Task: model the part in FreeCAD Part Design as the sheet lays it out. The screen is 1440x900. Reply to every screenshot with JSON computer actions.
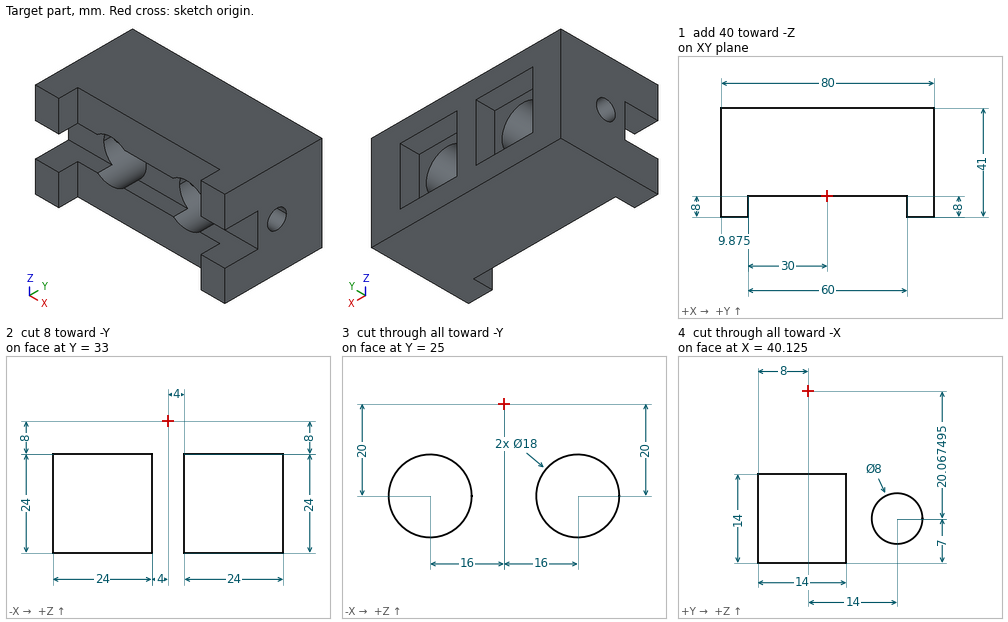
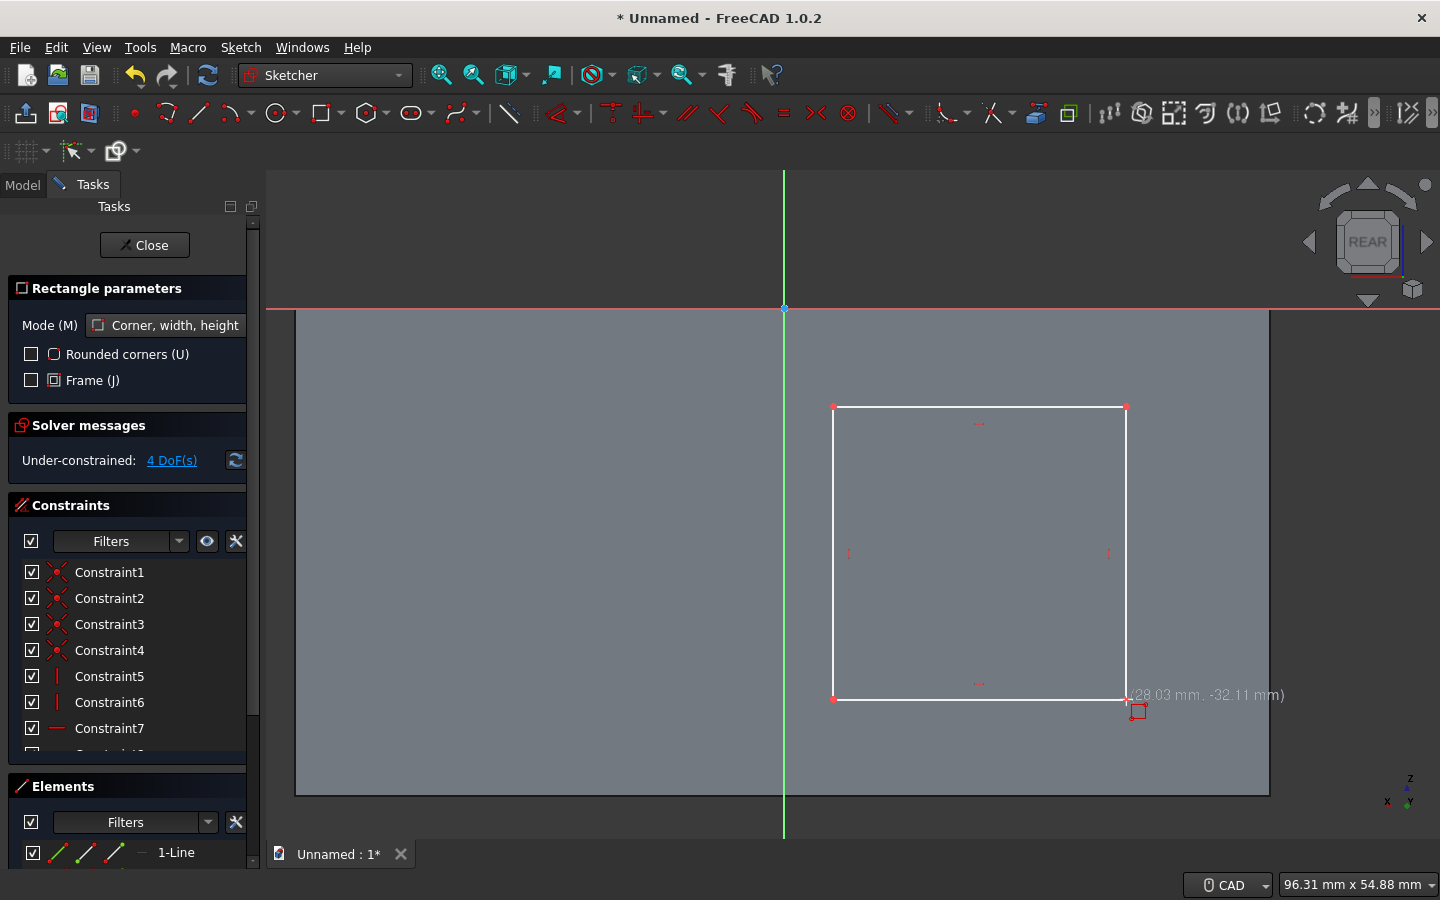
{"action": "left_click", "coordinate": [443, 406]}
{"action": "left_click", "coordinate": [736, 699]}
{"action": "key", "text": "Escape"}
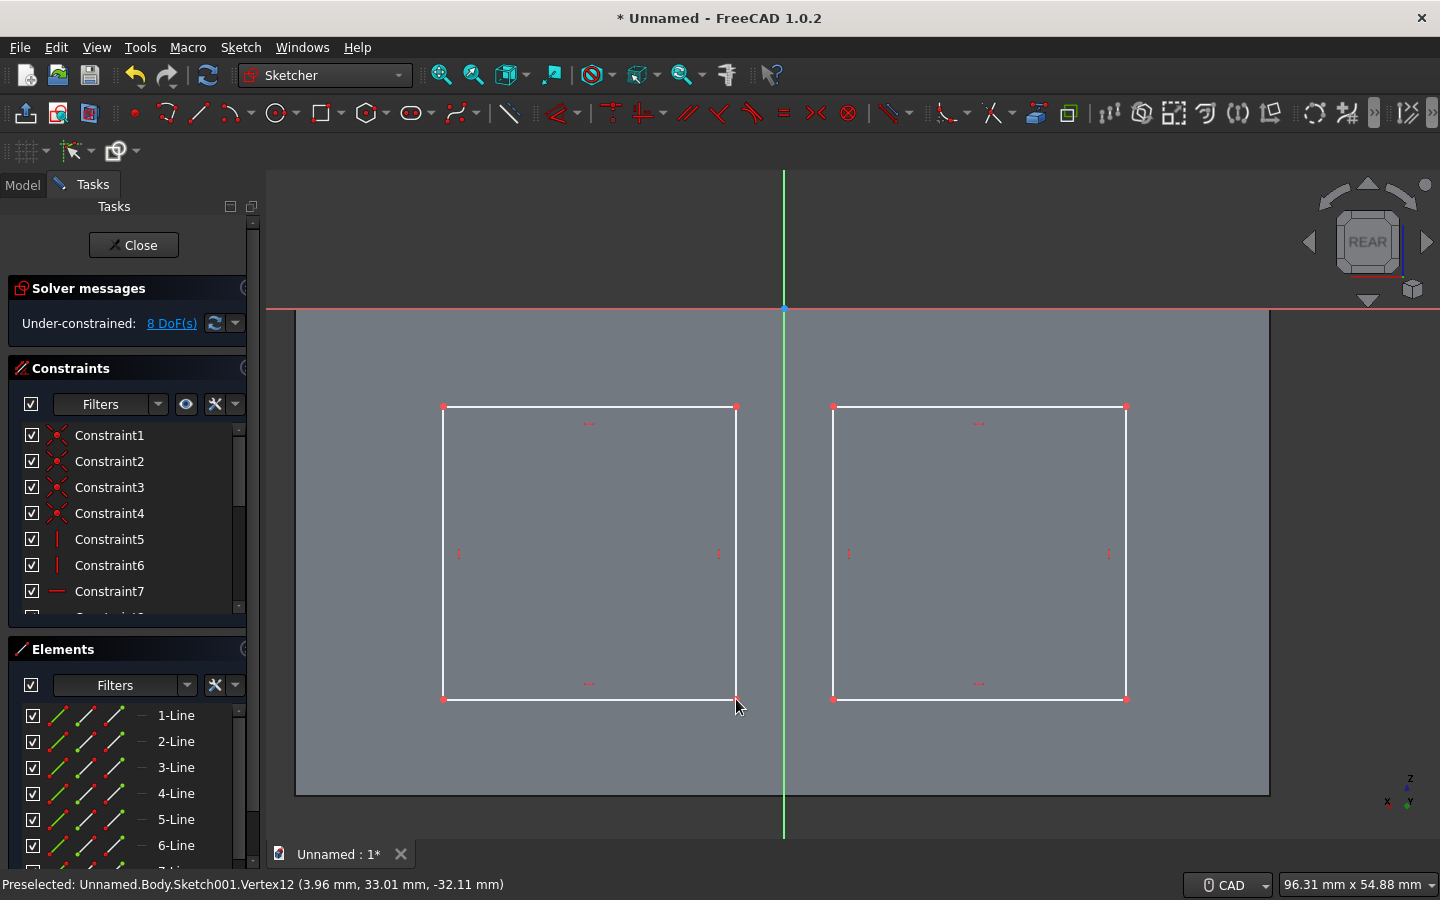
{"action": "left_click", "coordinate": [556, 114]}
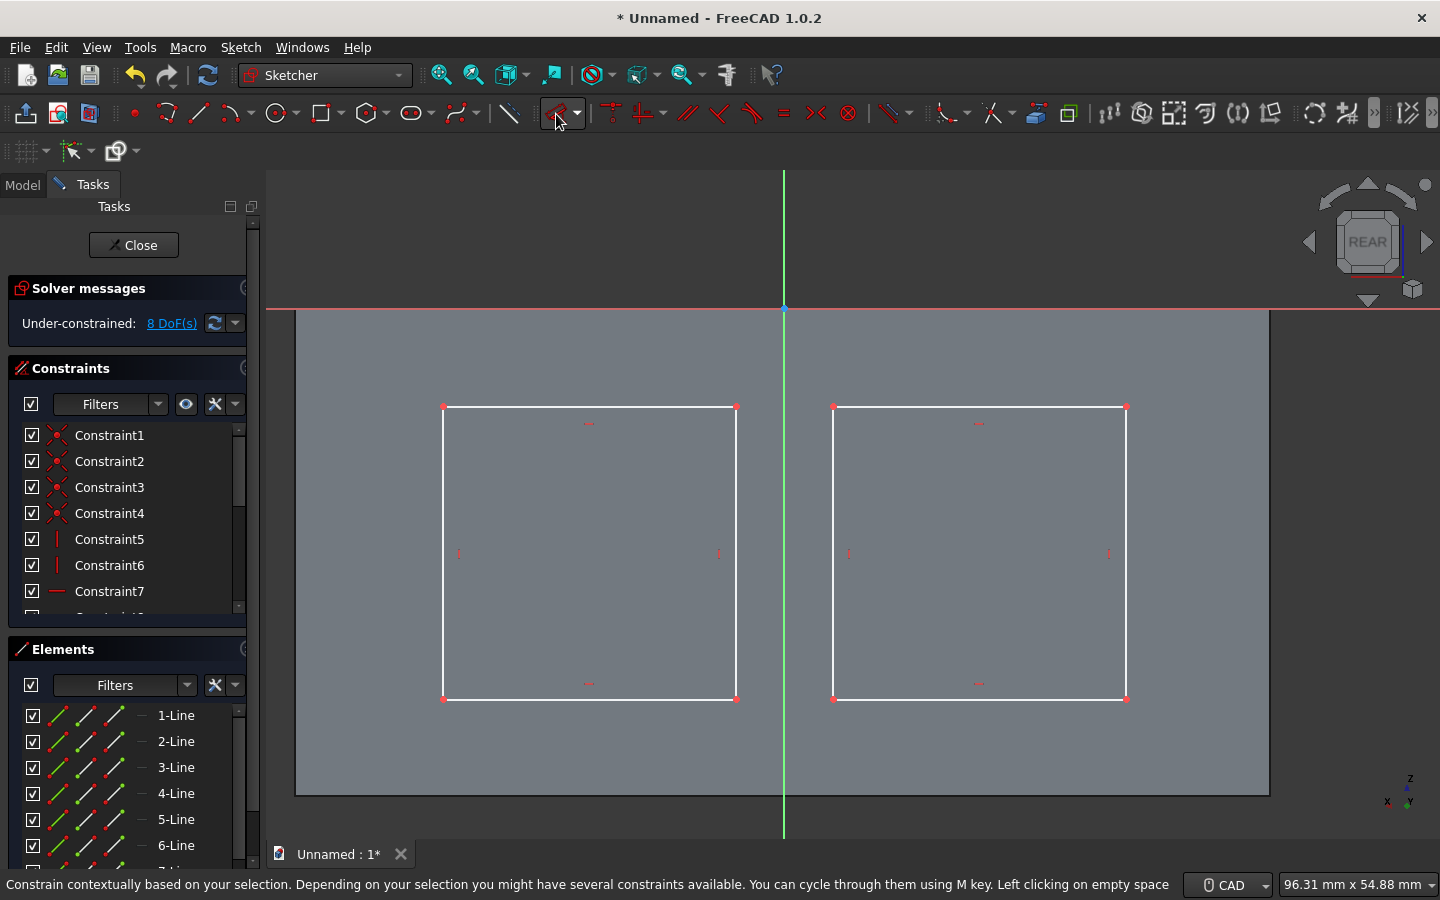
{"action": "left_click", "coordinate": [833, 495]}
{"action": "left_click", "coordinate": [867, 553]}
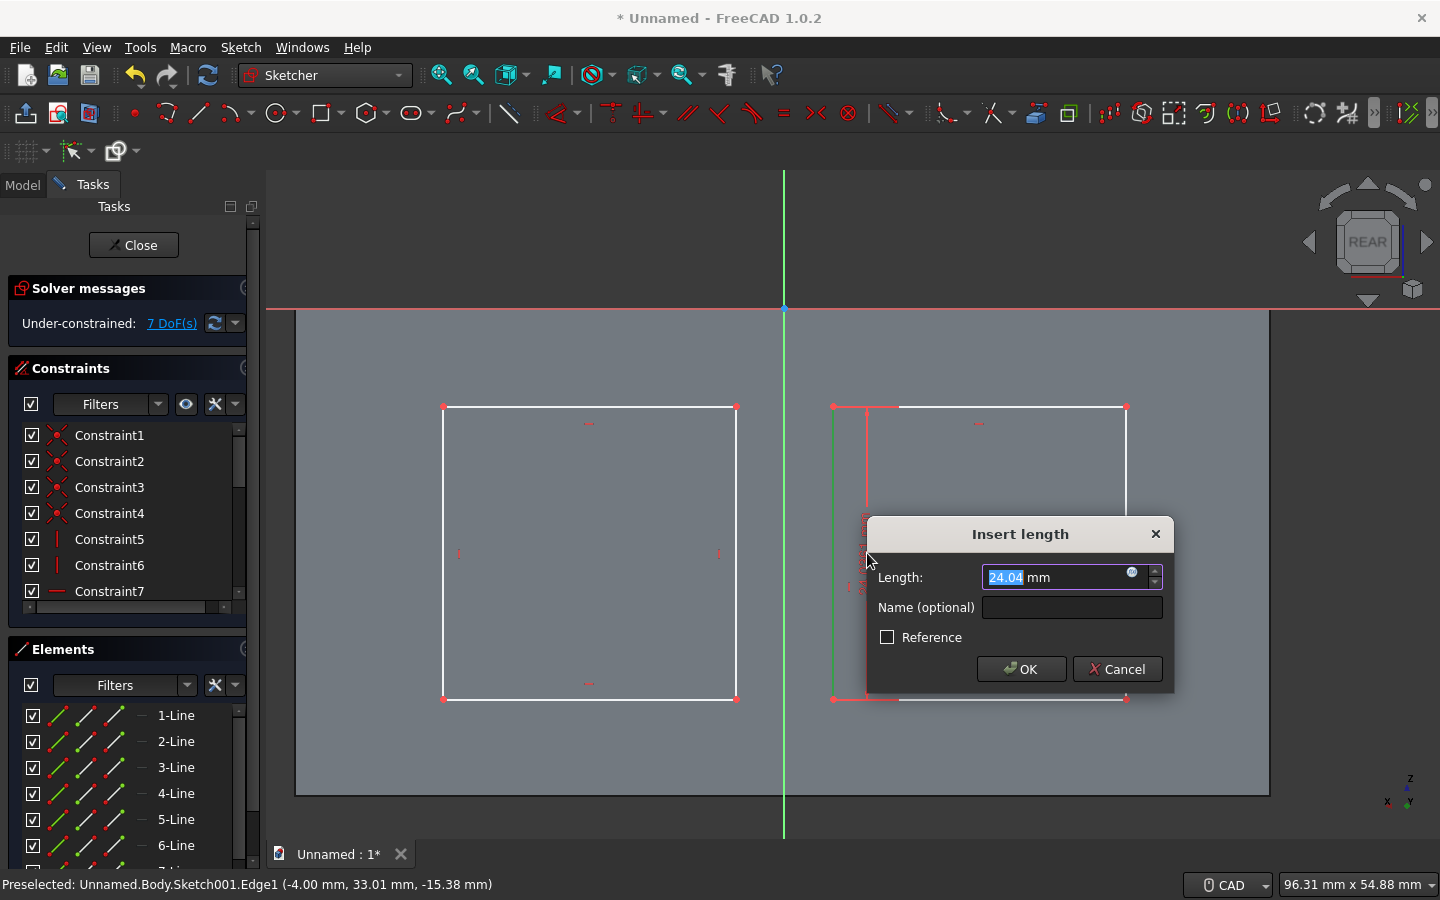
{"action": "type", "text": "24"}
{"action": "key", "text": "Return"}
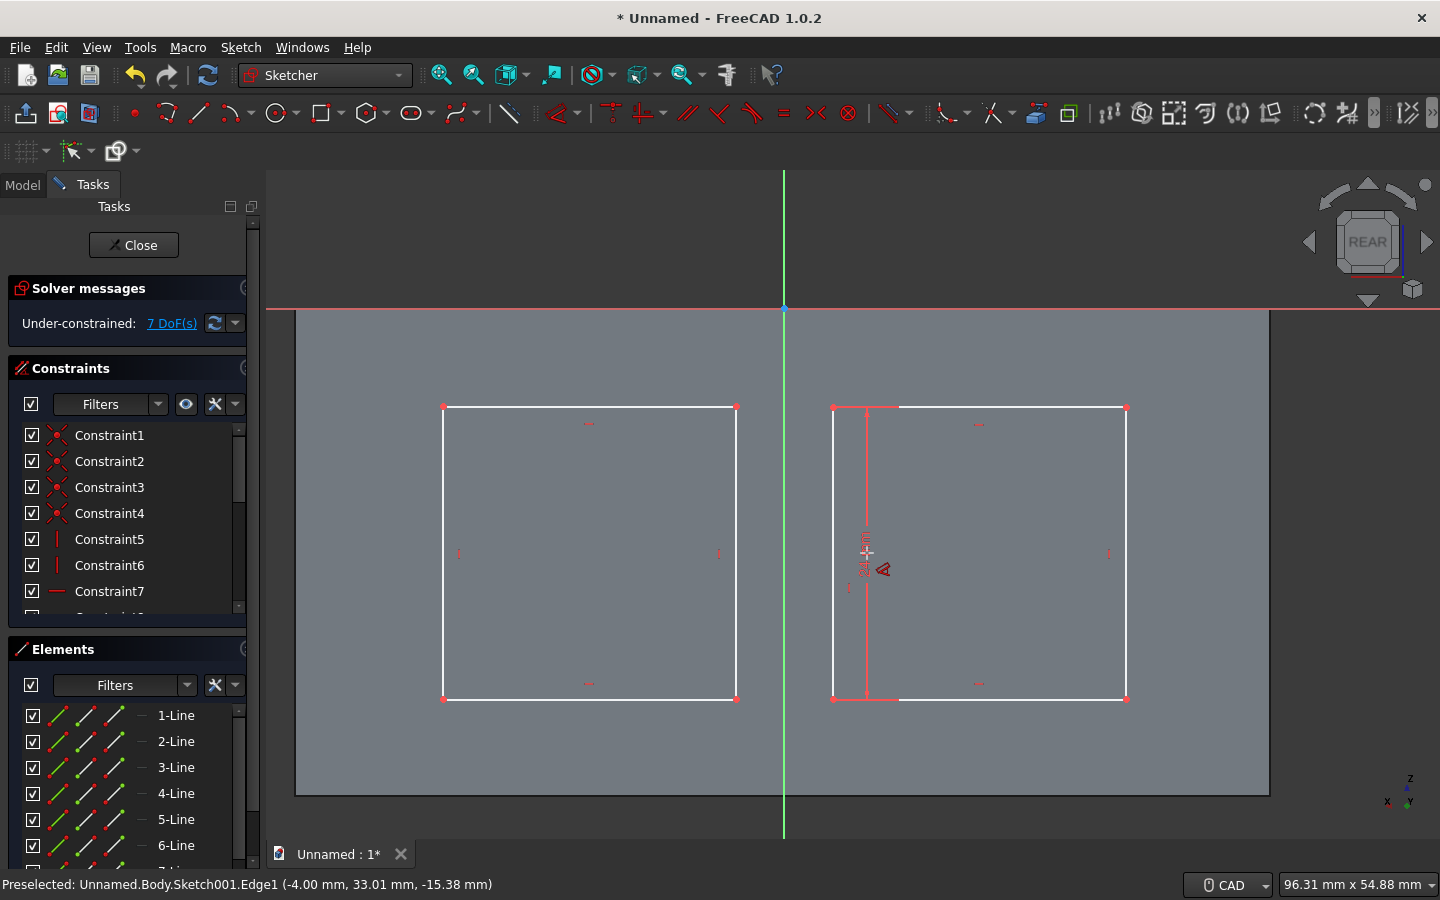
{"action": "left_click", "coordinate": [921, 700]}
{"action": "left_click", "coordinate": [979, 734]}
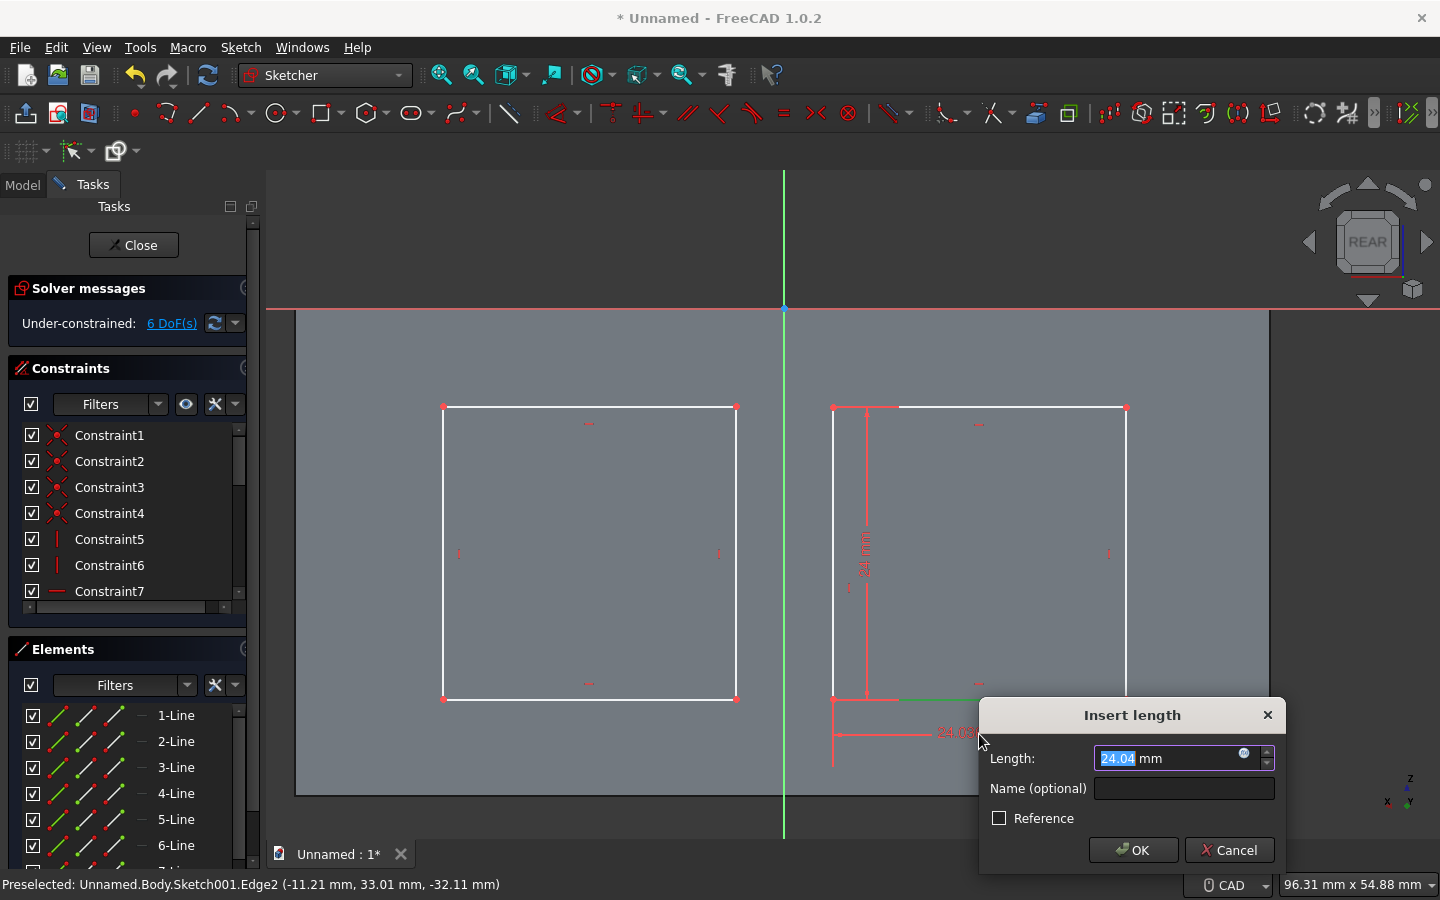
{"action": "type", "text": "24"}
{"action": "key", "text": "Return"}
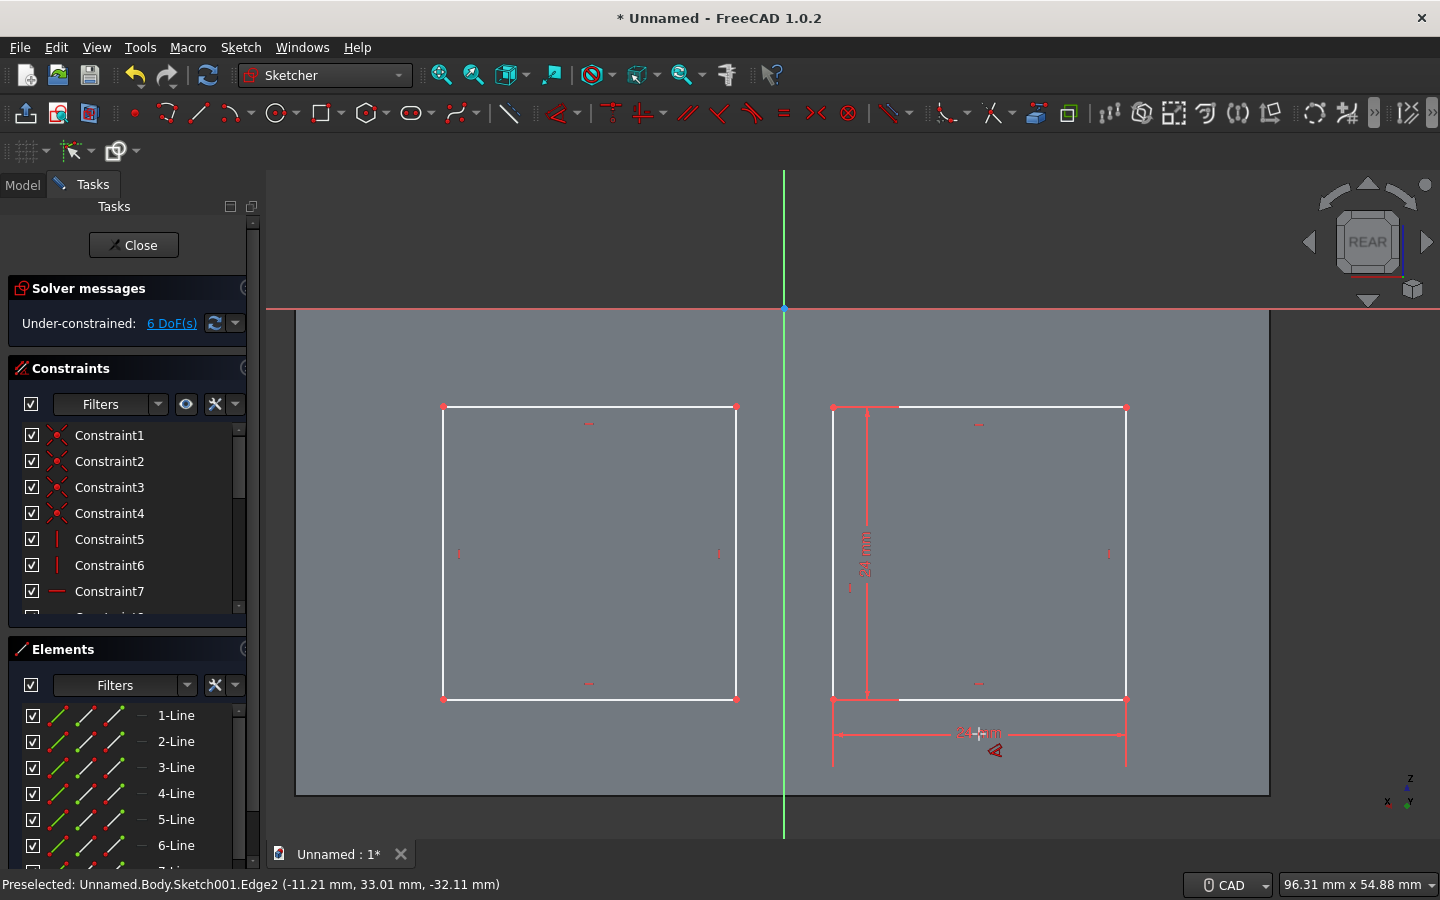
{"action": "left_click", "coordinate": [443, 495]}
{"action": "left_click", "coordinate": [409, 553]}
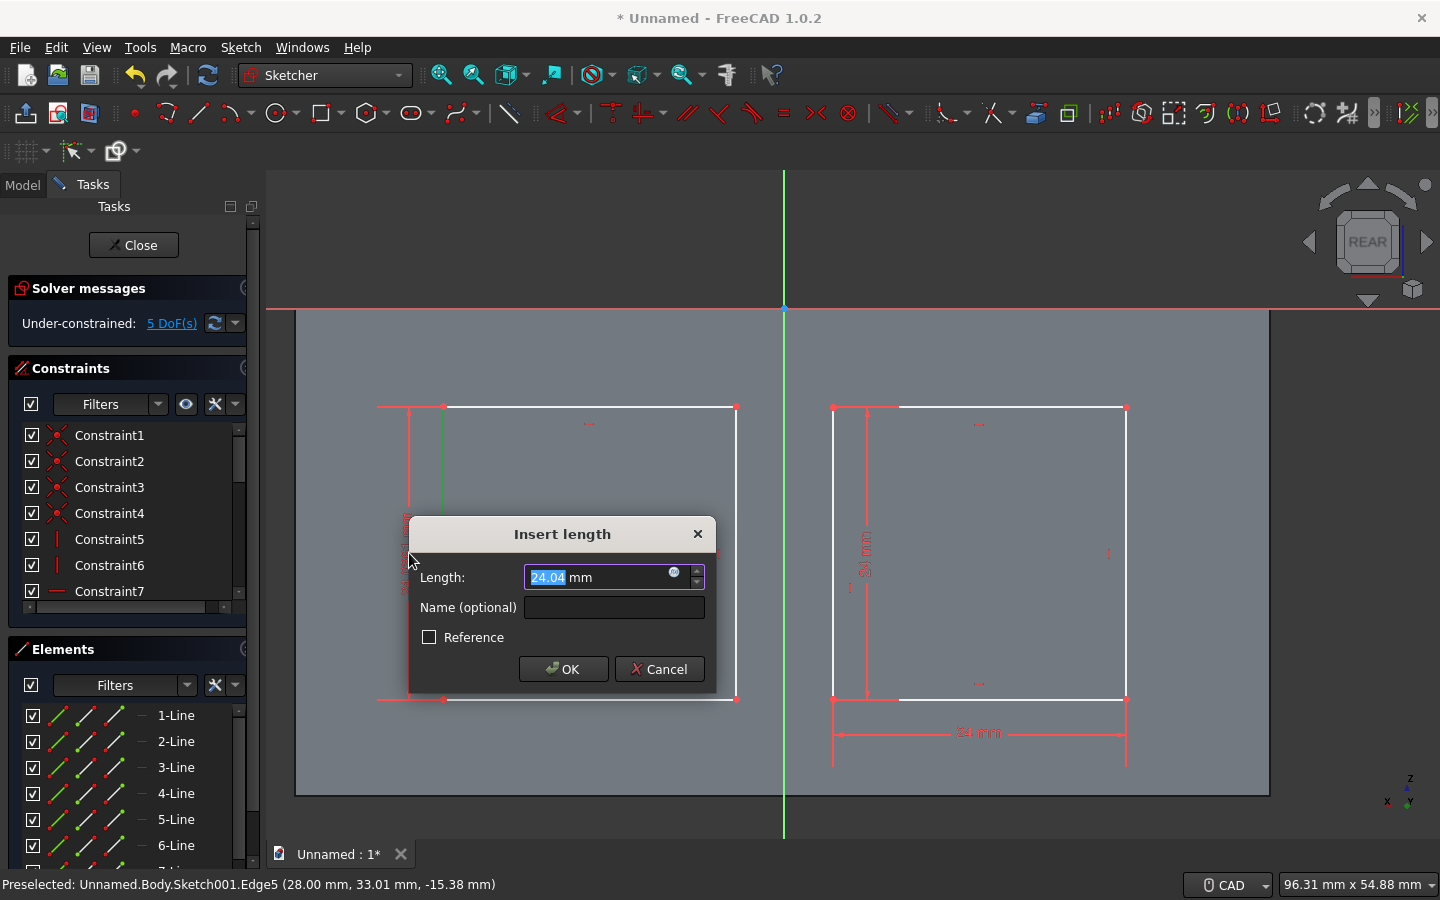
{"action": "type", "text": "24"}
{"action": "key", "text": "Return"}